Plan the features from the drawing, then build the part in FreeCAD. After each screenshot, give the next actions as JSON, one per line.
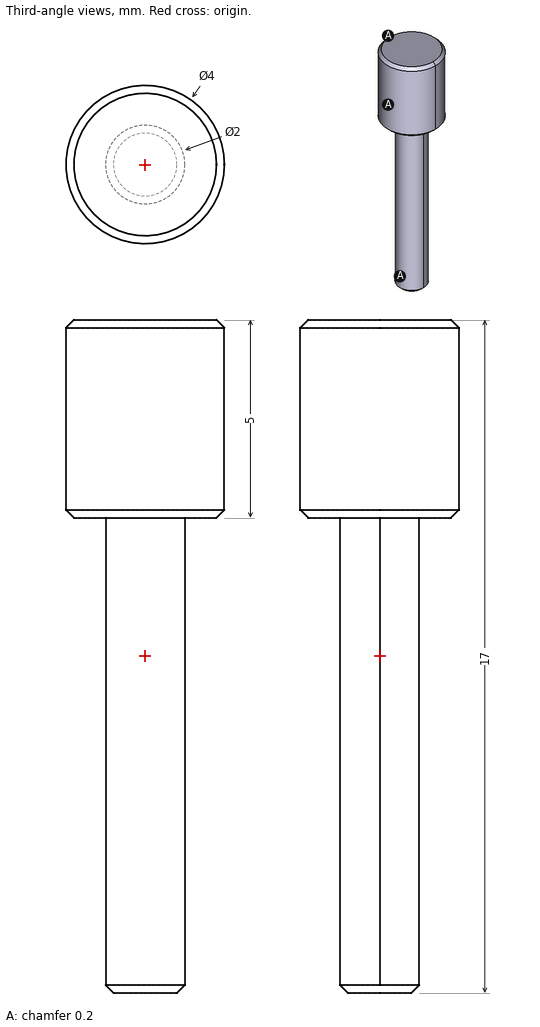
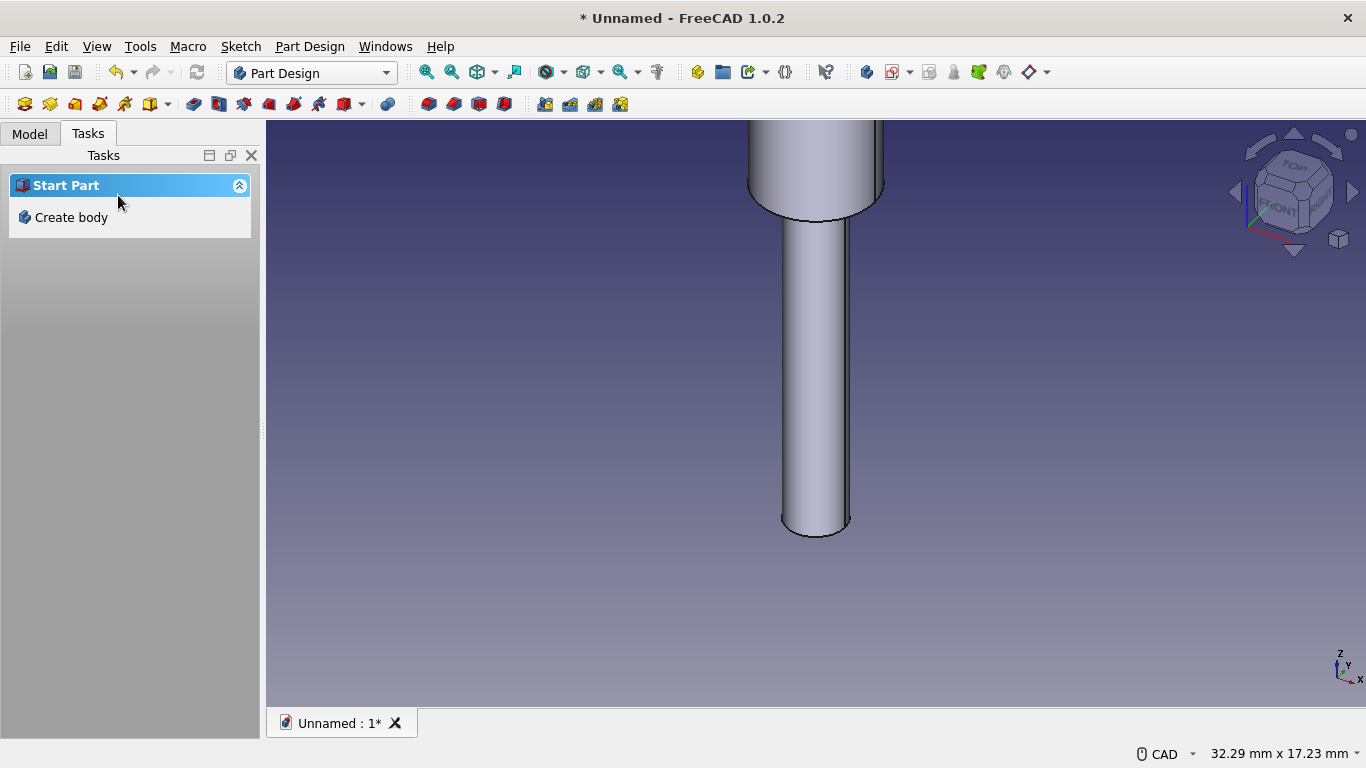
{"action": "left_click", "coordinate": [427, 72]}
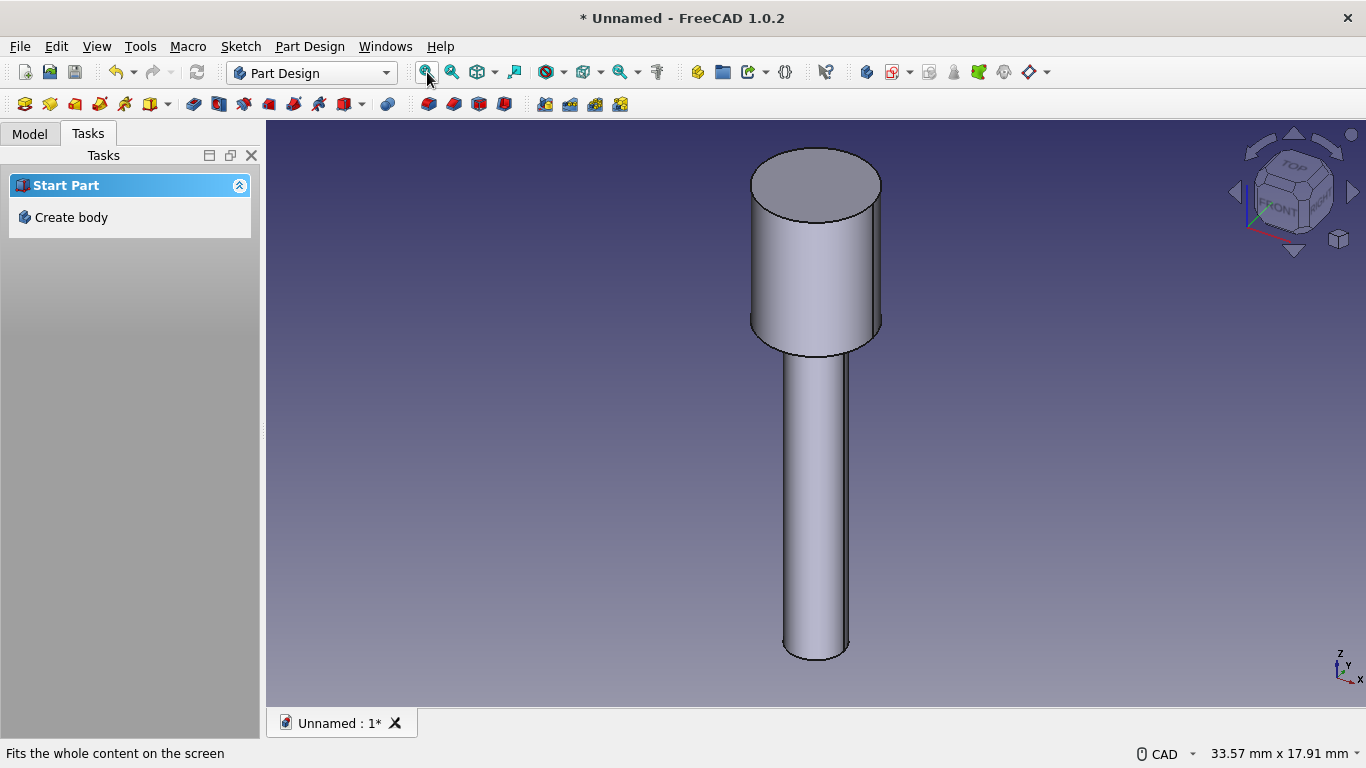
{"action": "left_click", "coordinate": [751, 188]}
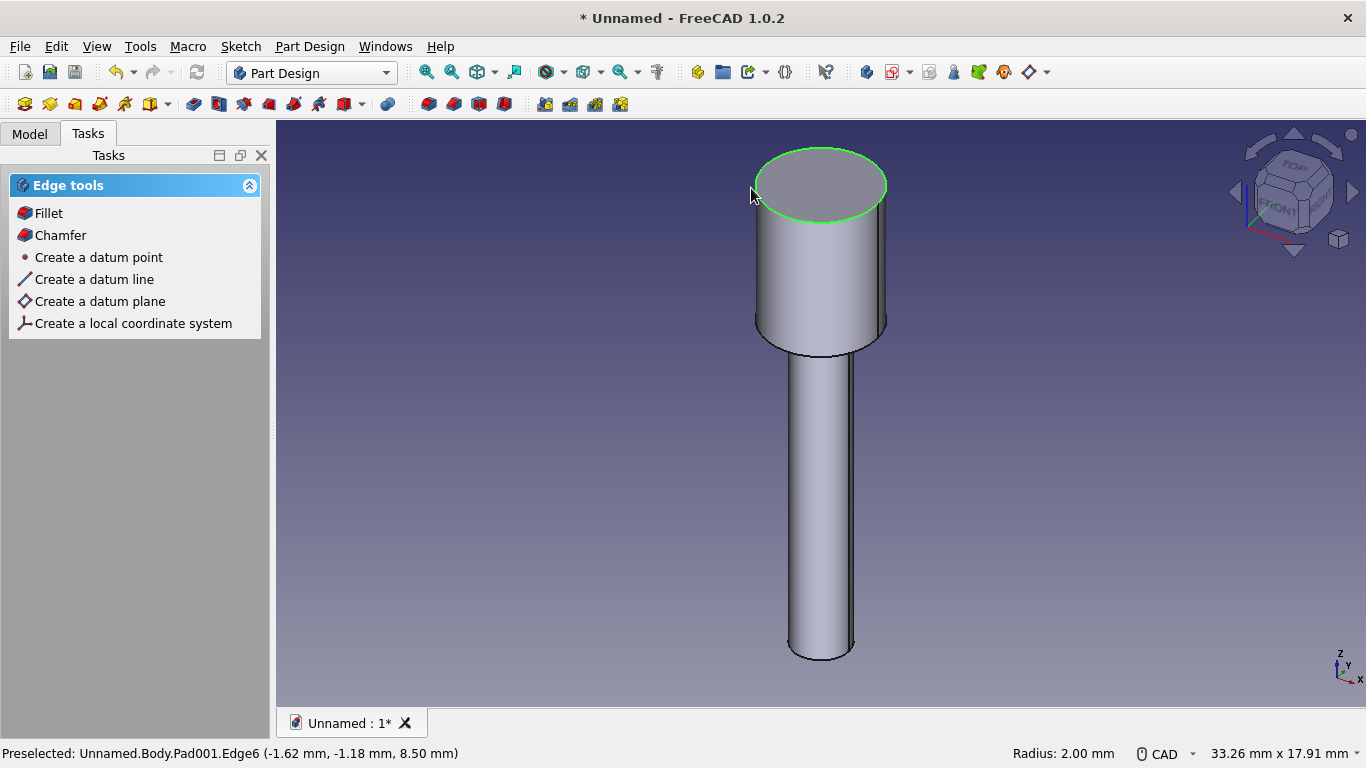
{"action": "key", "text": "0"}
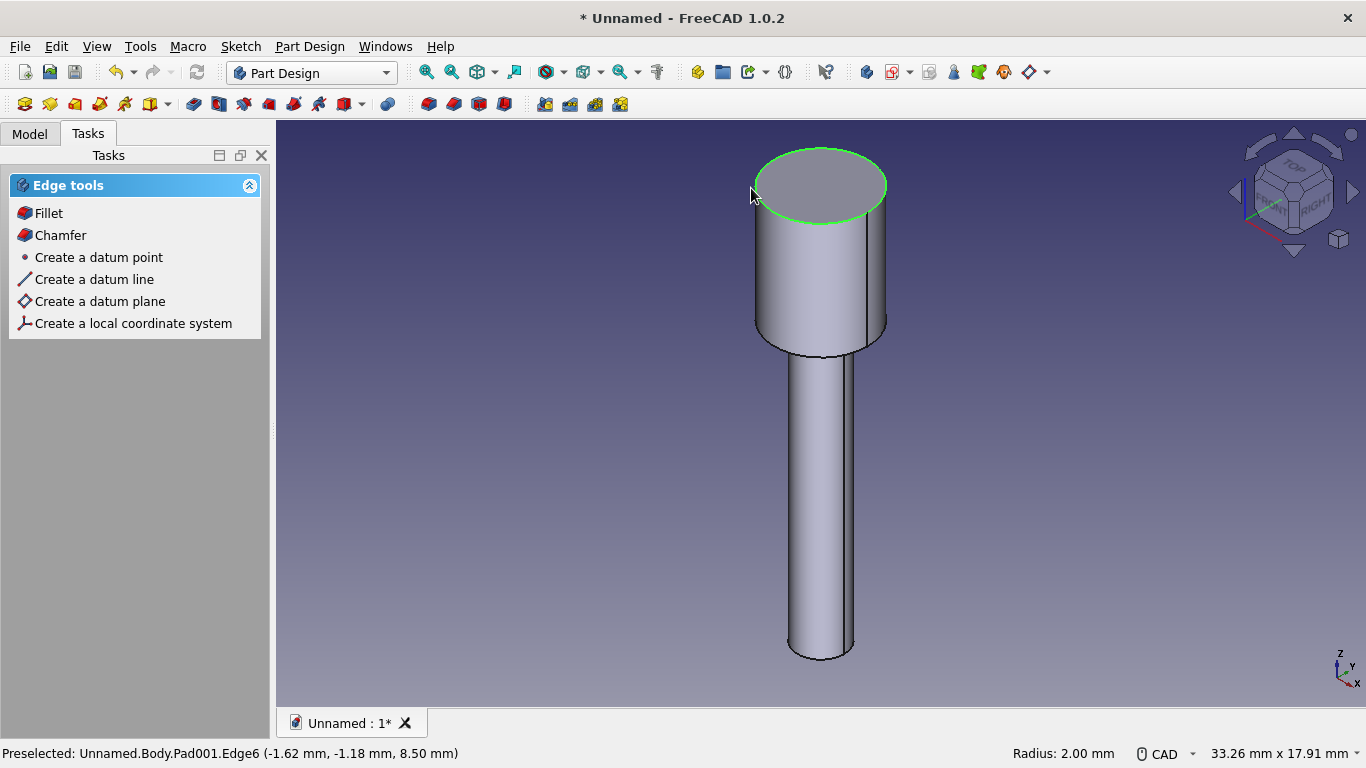
{"action": "key", "text": "2"}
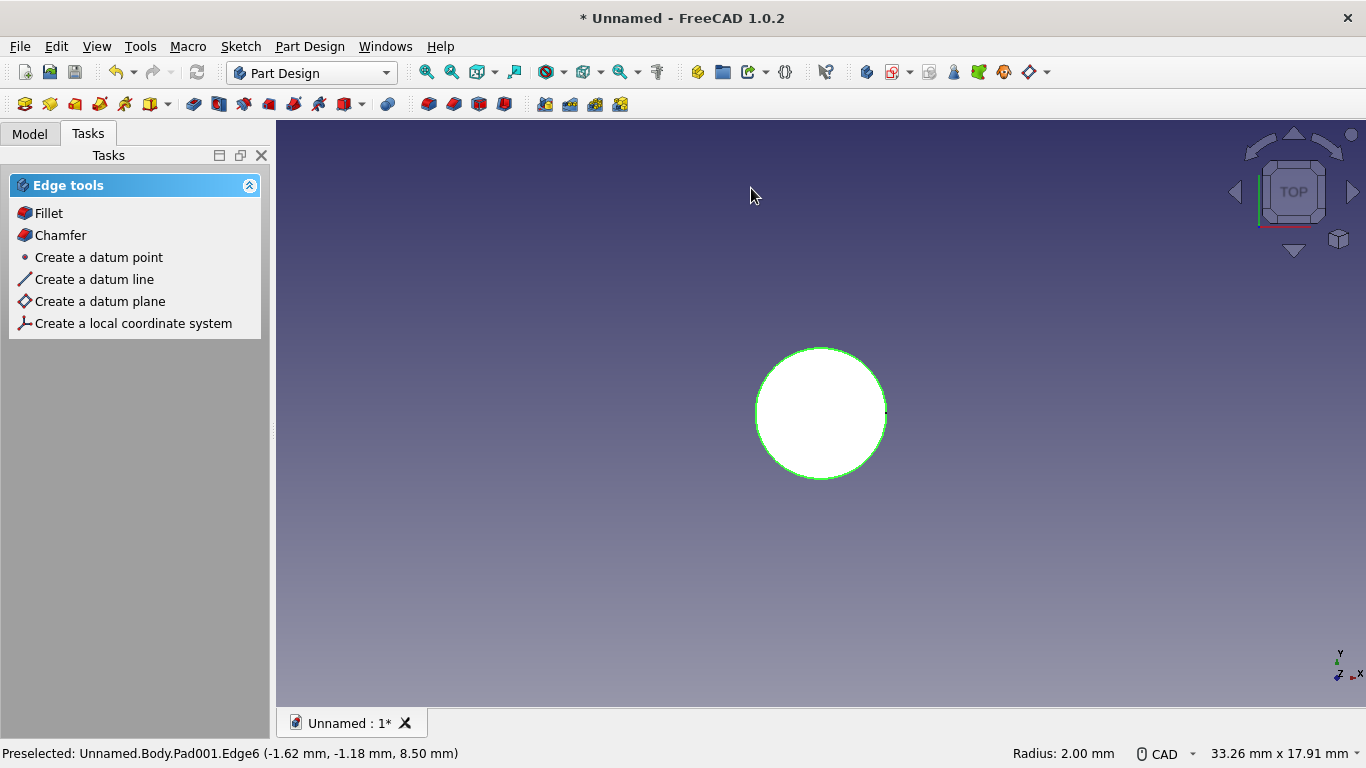
{"action": "left_click", "coordinate": [427, 72]}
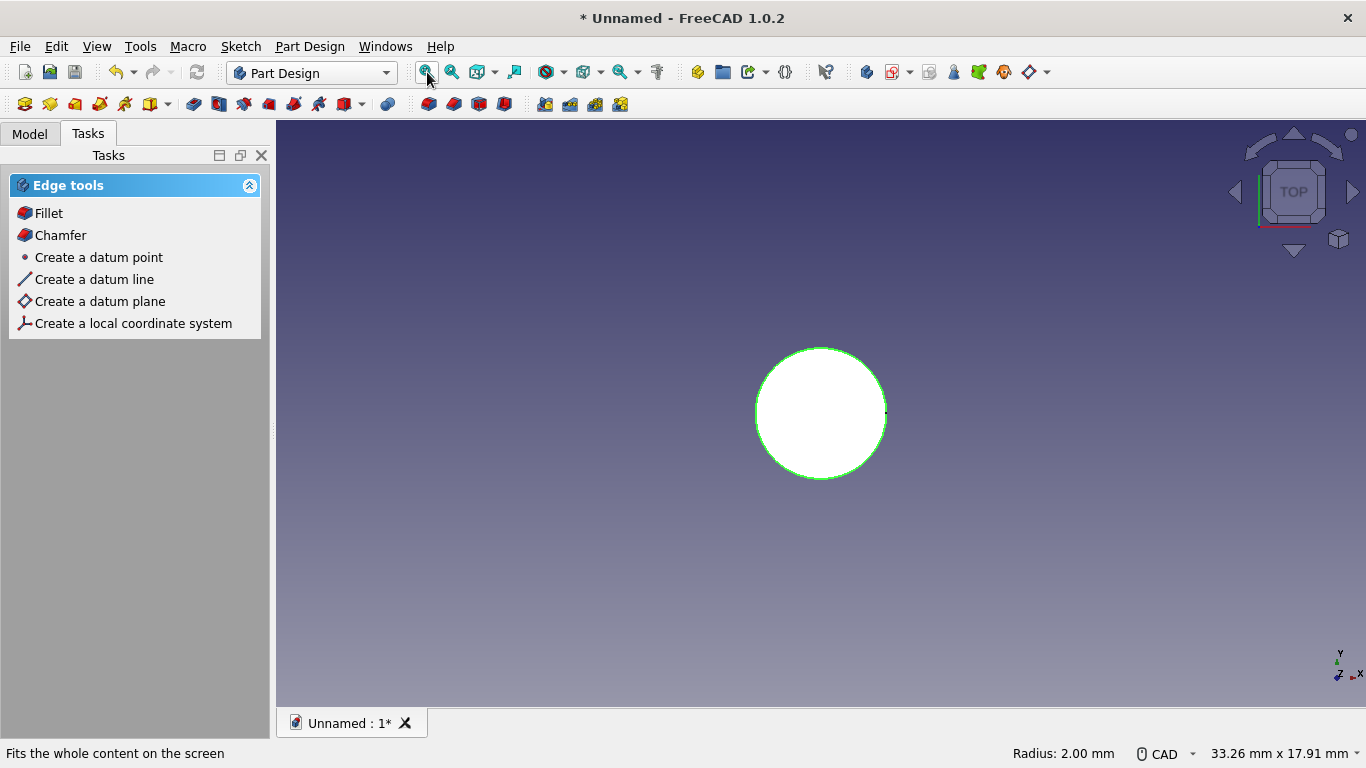
{"action": "key", "text": "1"}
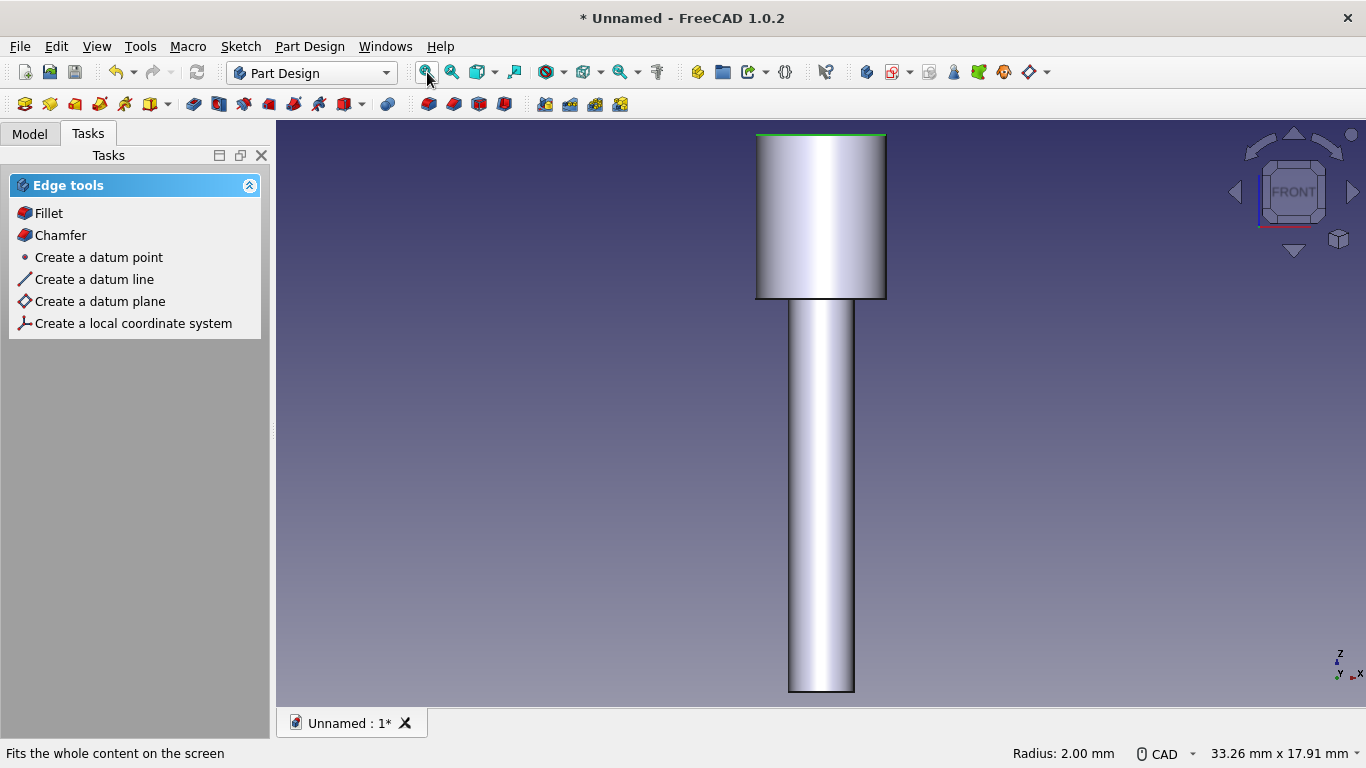
{"action": "left_click", "coordinate": [768, 298], "text": "ctrl"}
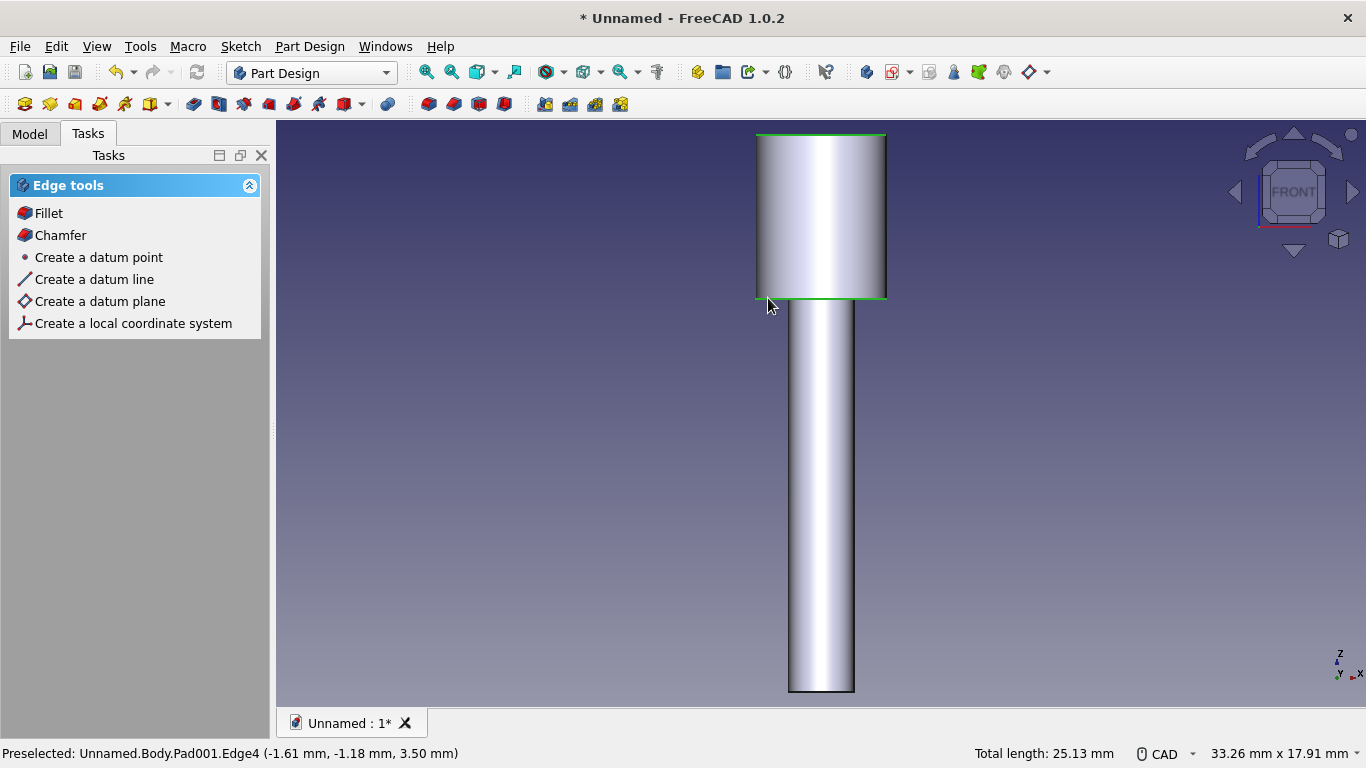
{"action": "key", "text": "3"}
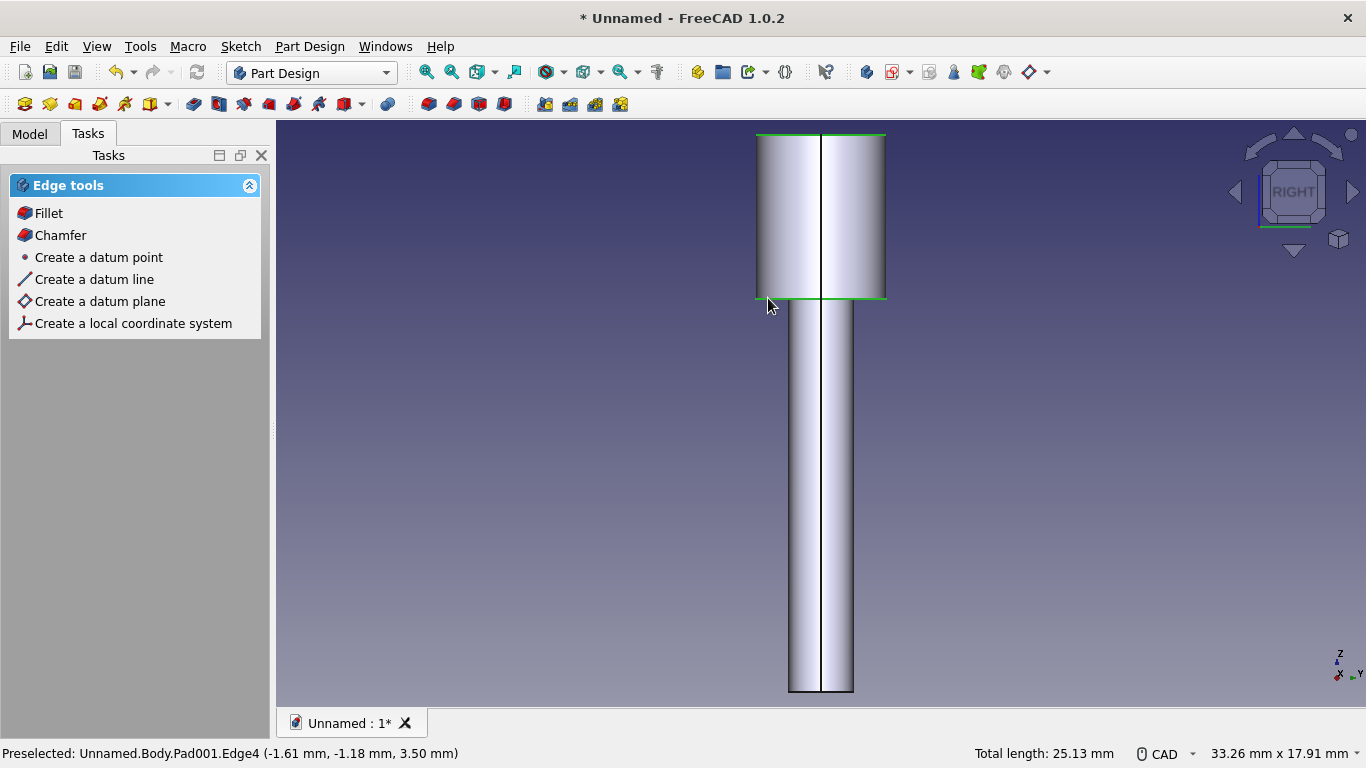
{"action": "key", "text": "5"}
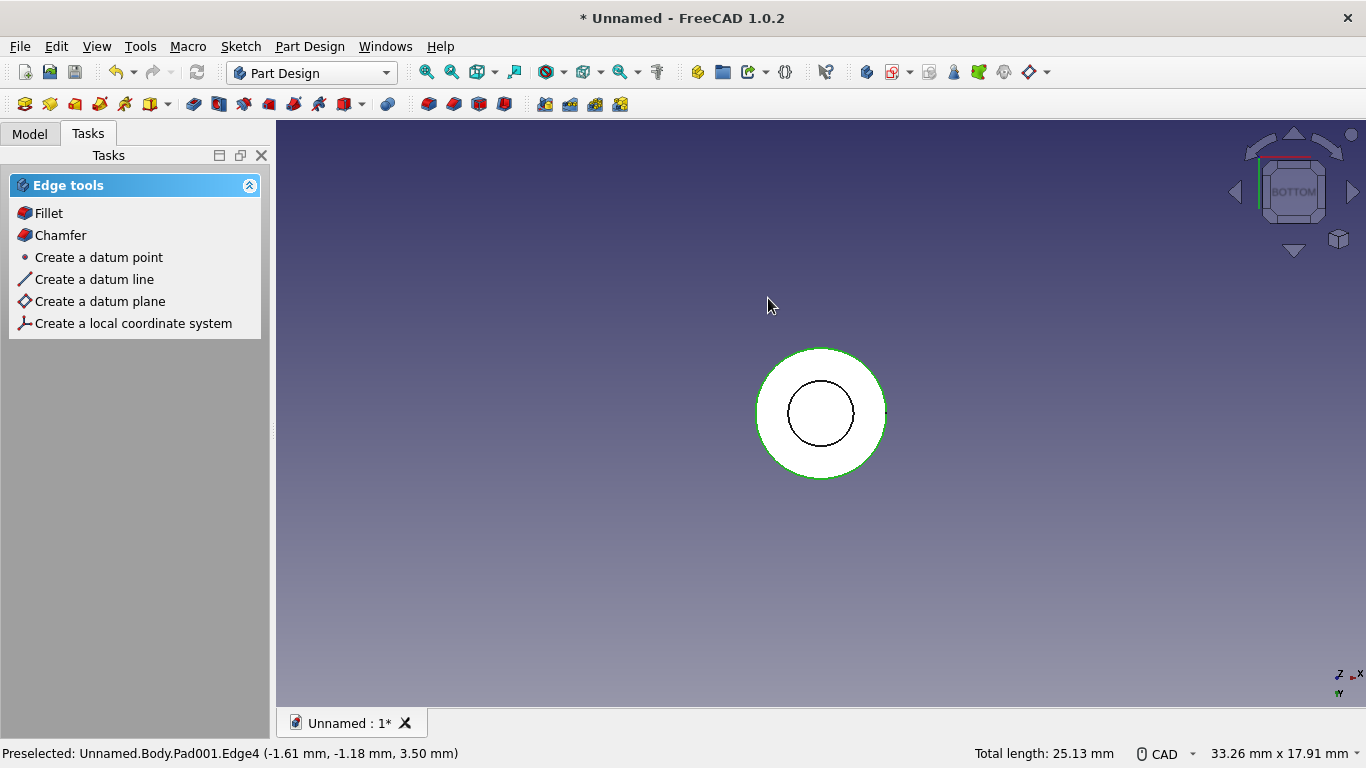
{"action": "left_click", "coordinate": [427, 72]}